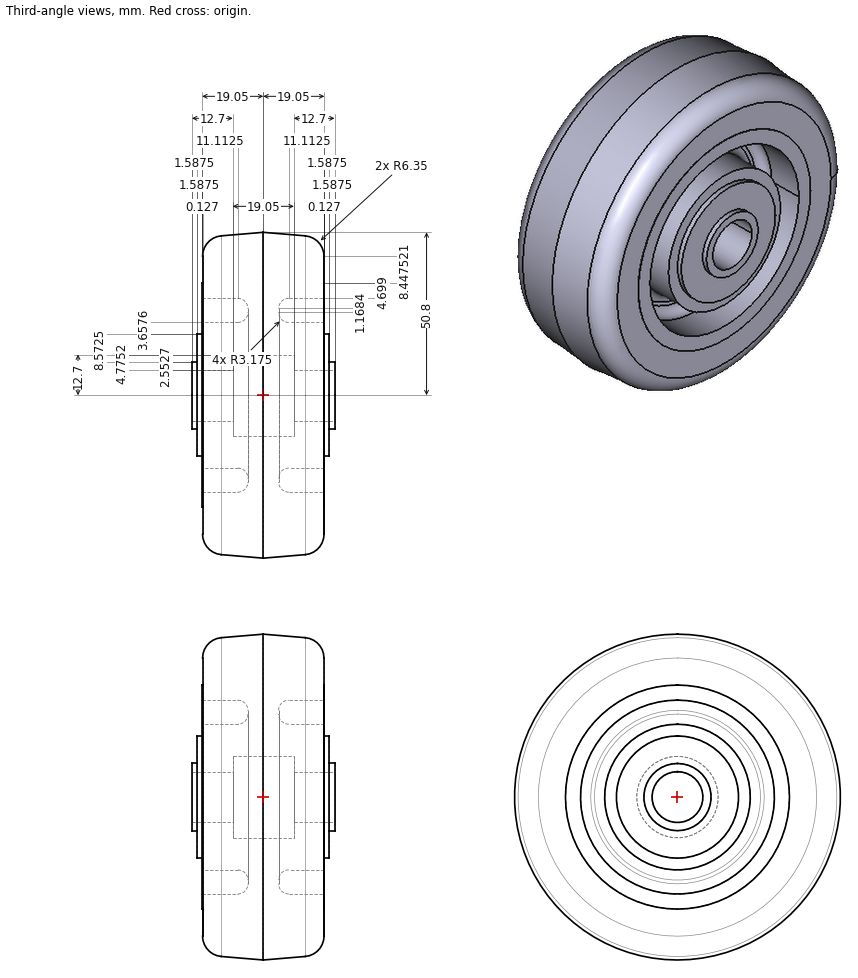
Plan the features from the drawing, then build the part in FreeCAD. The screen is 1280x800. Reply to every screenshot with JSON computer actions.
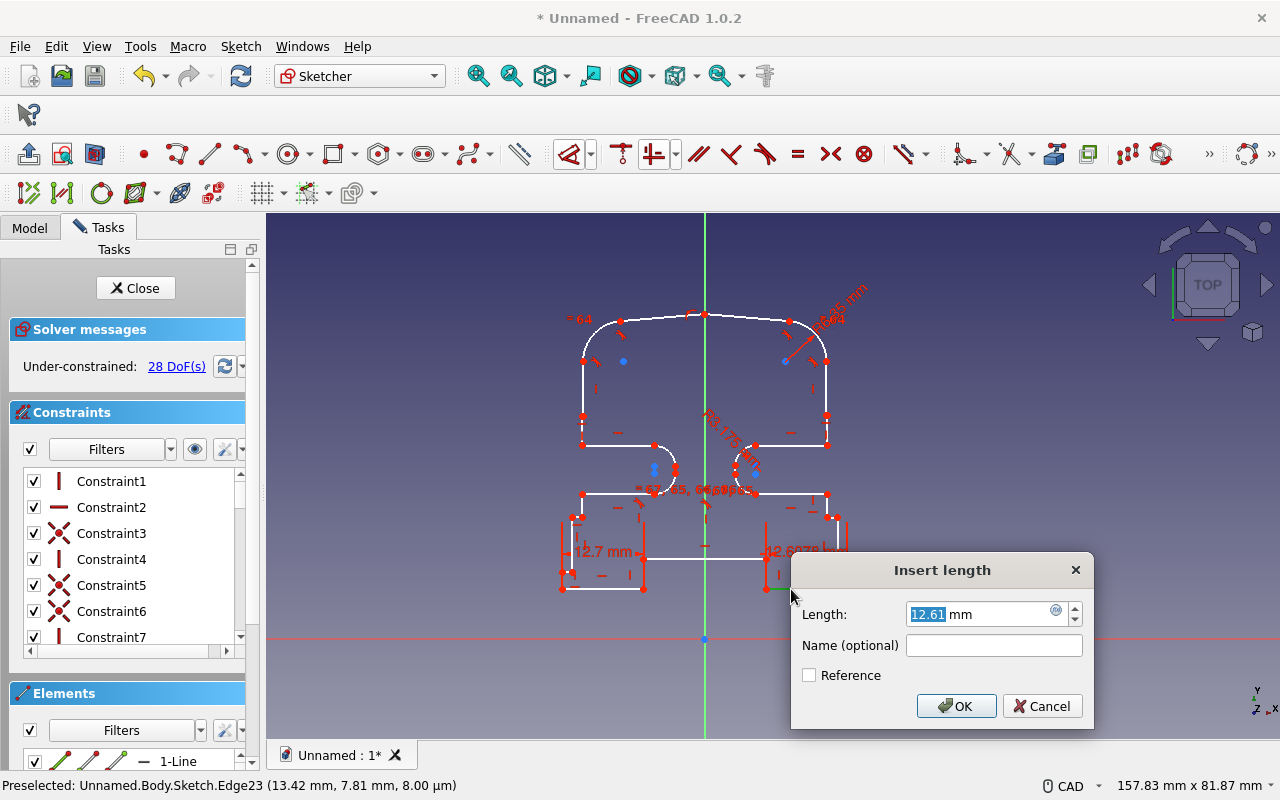
{"action": "type", "text": "12.7"}
{"action": "key", "text": "Return"}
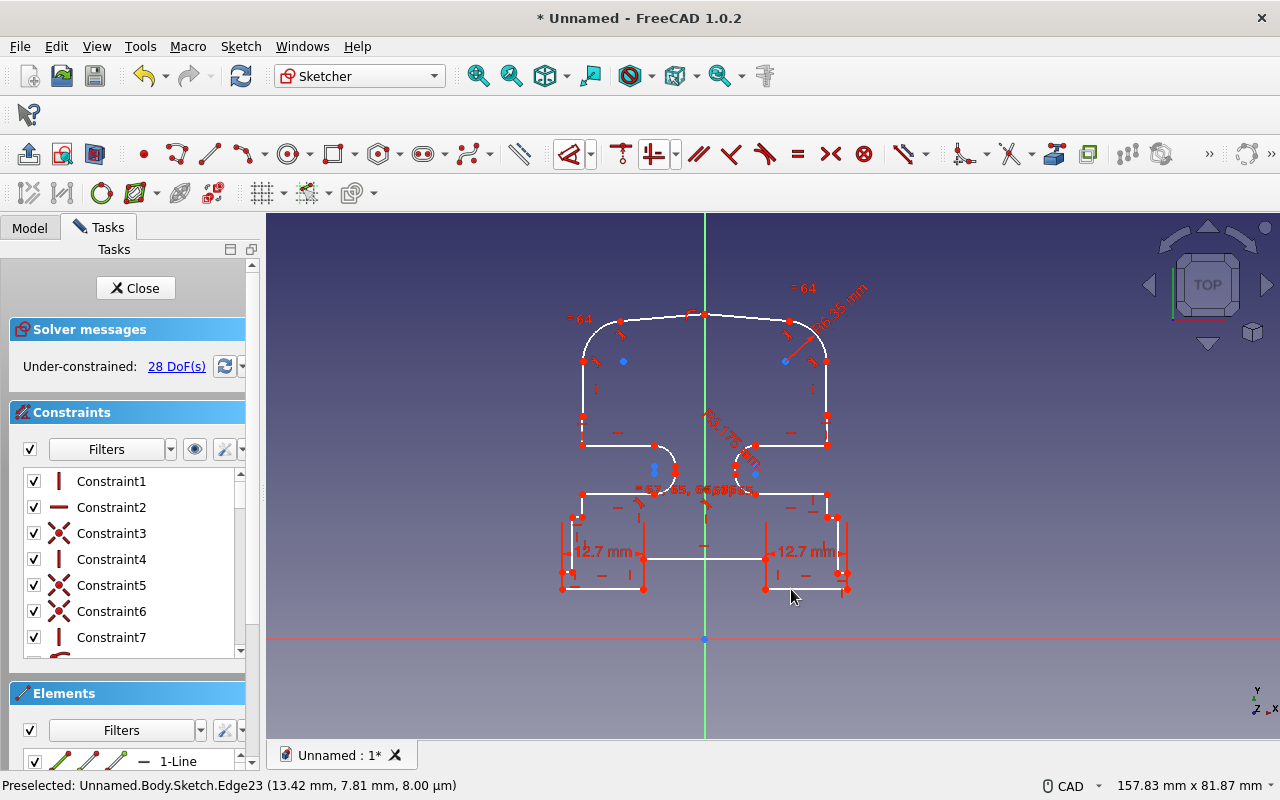
{"action": "scroll", "coordinate": [827, 434], "scroll_direction": "up", "scroll_amount": 2}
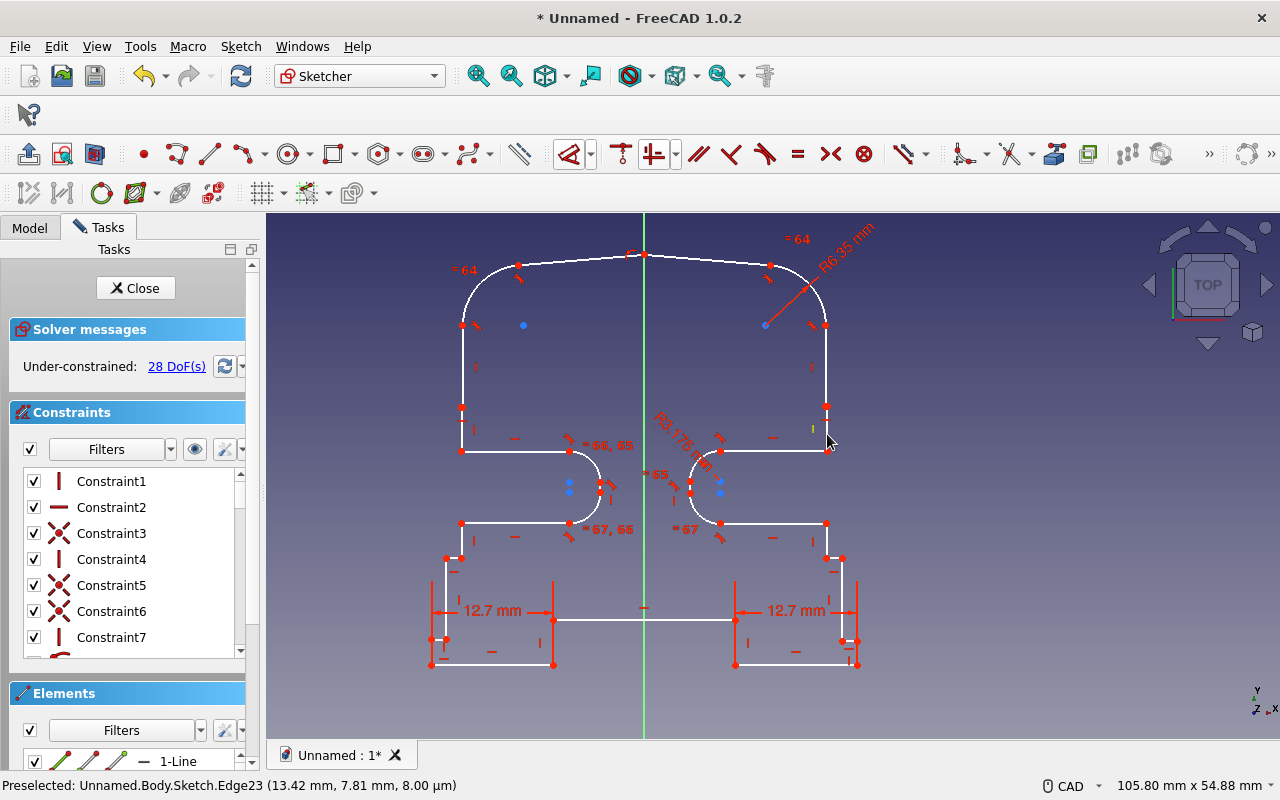
{"action": "left_click", "coordinate": [827, 433]}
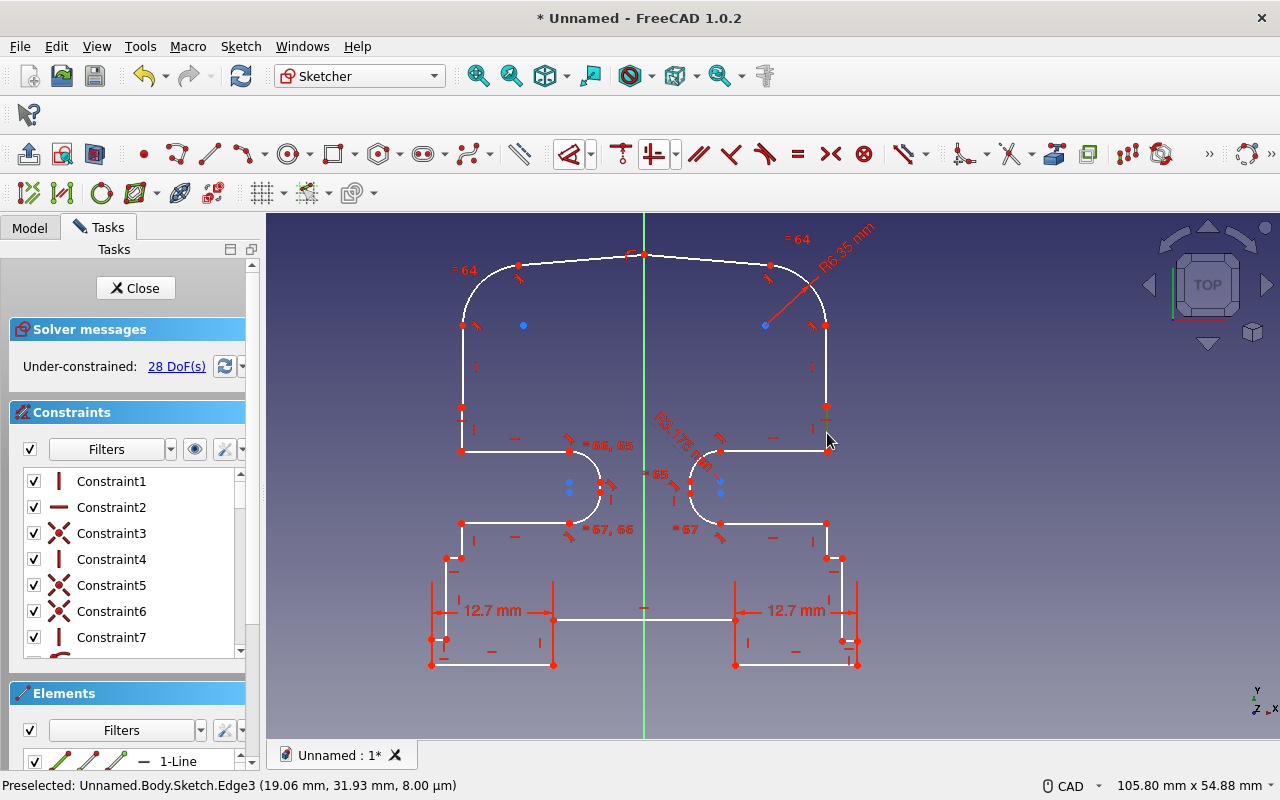
{"action": "key", "text": "i"}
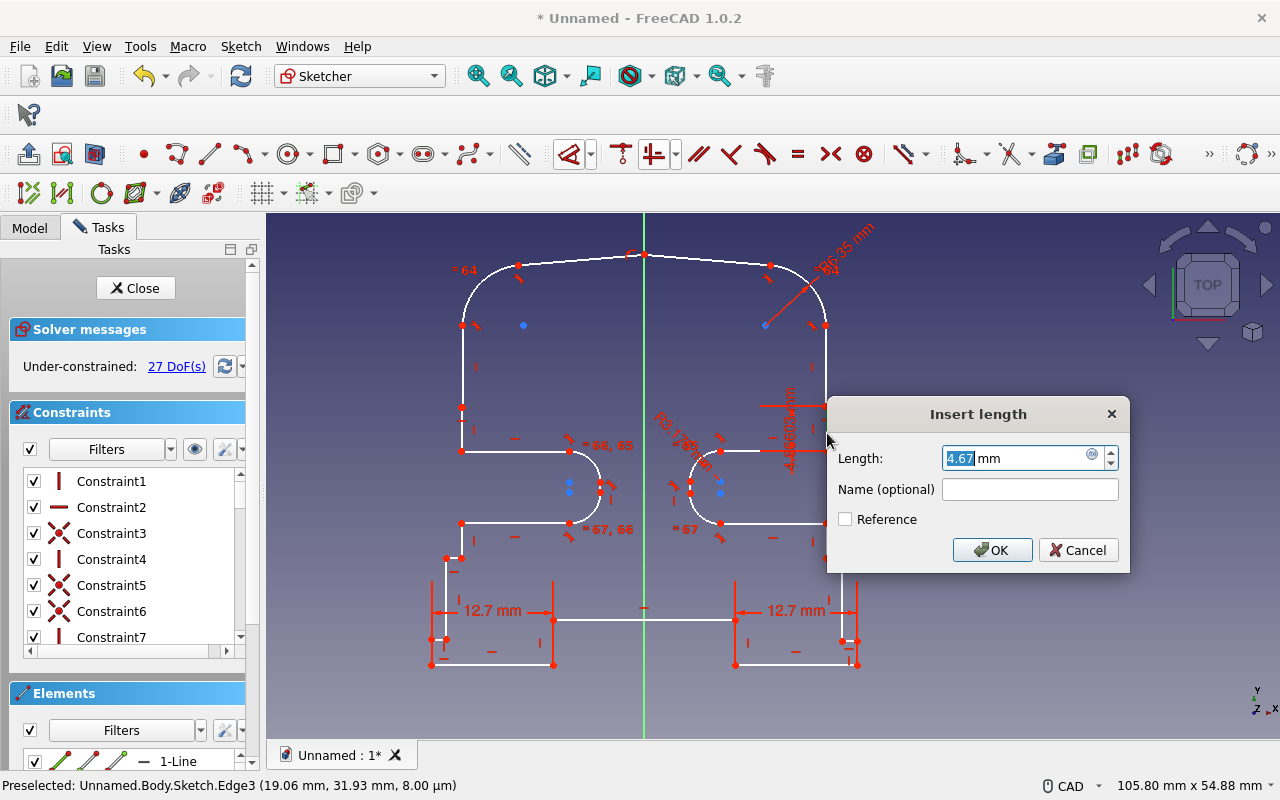
{"action": "type", "text": "4.699"}
{"action": "key", "text": "Return"}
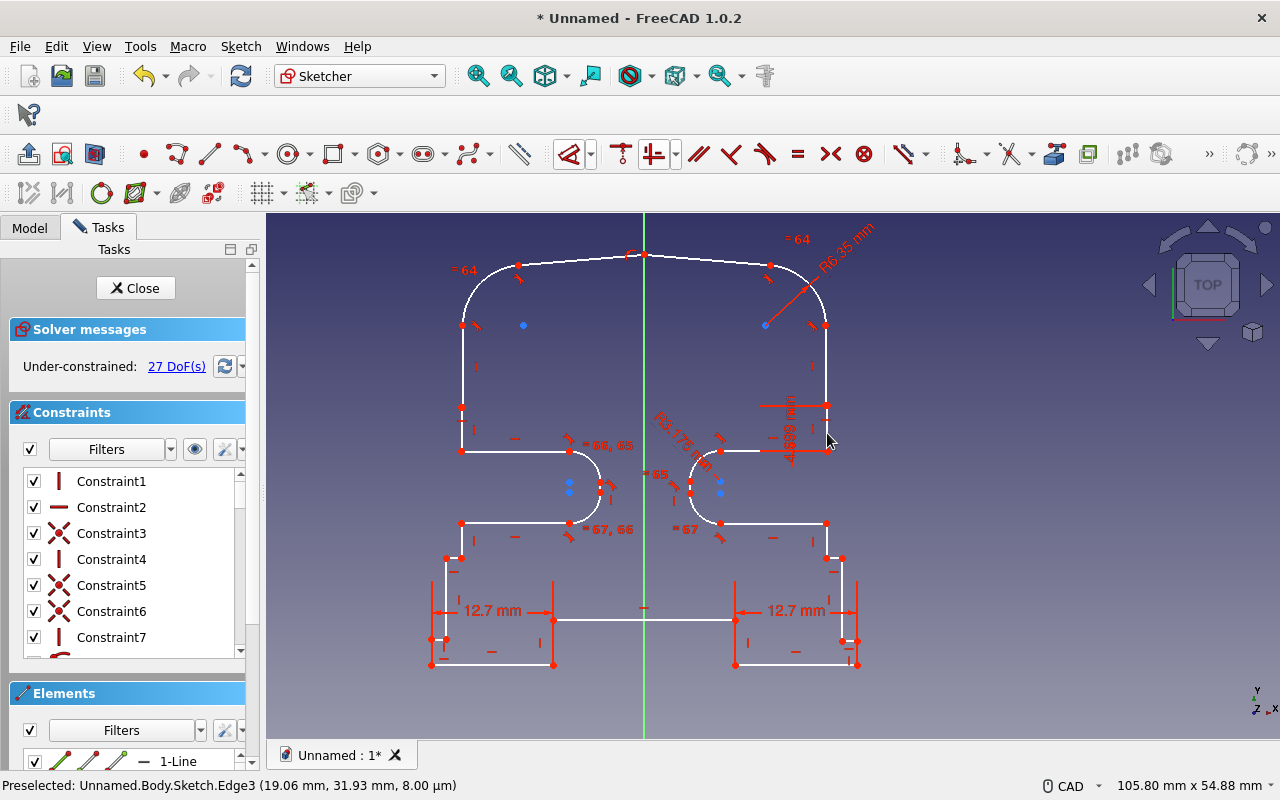
{"action": "scroll", "coordinate": [826, 406], "scroll_direction": "up", "scroll_amount": 18}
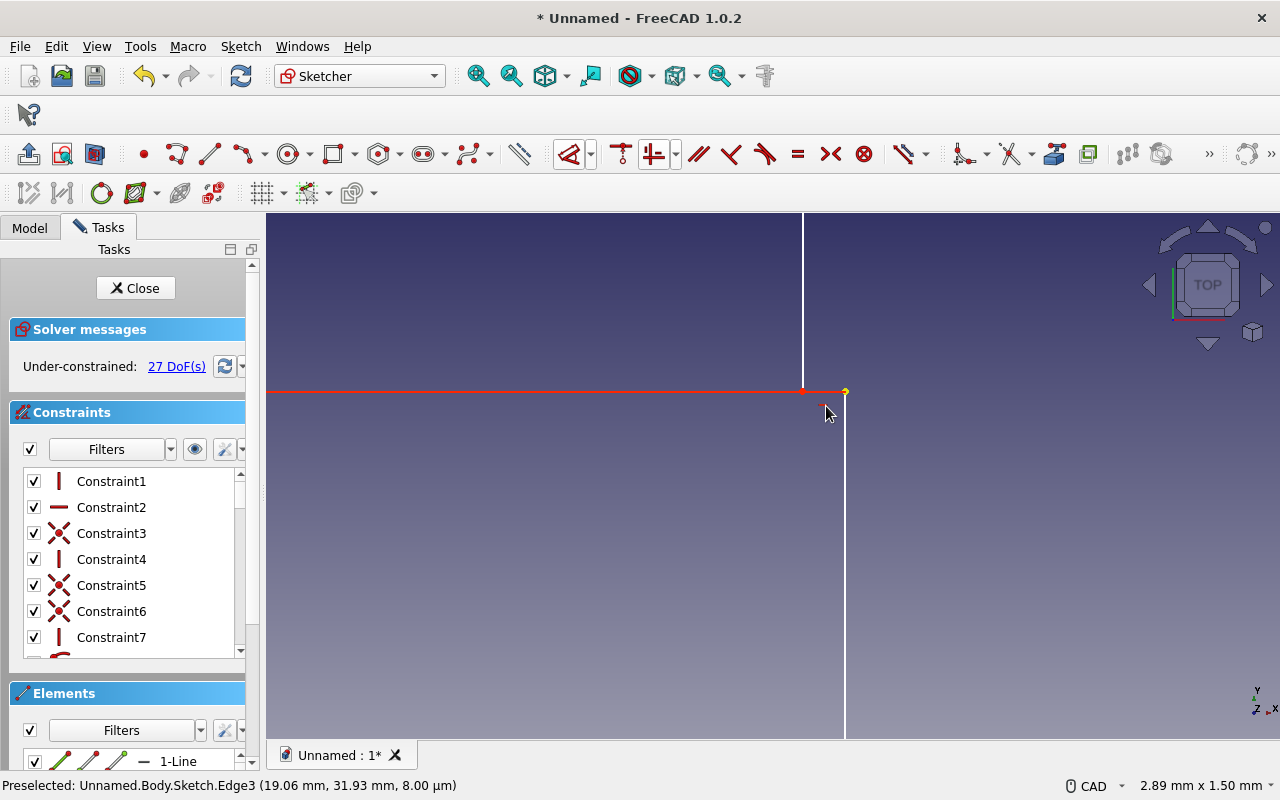
{"action": "left_click", "coordinate": [824, 392]}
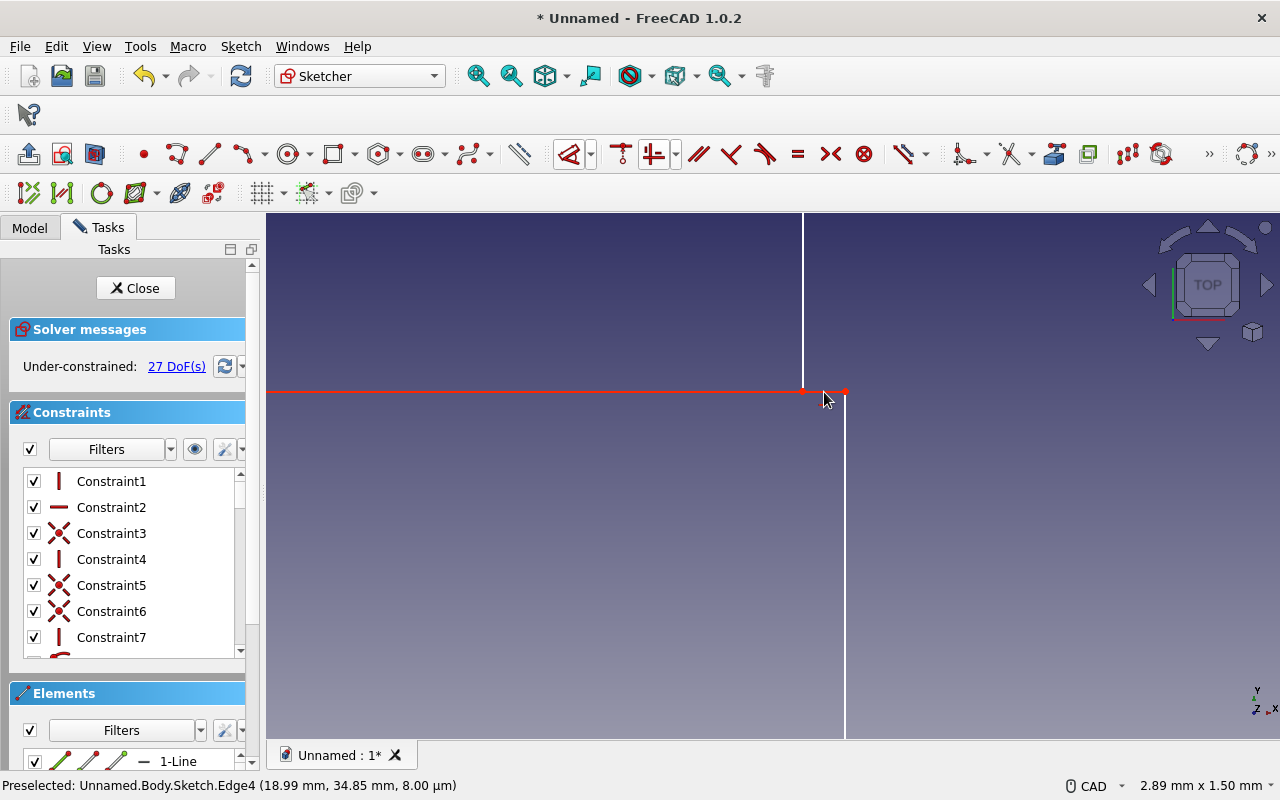
{"action": "left_click", "coordinate": [590, 154]}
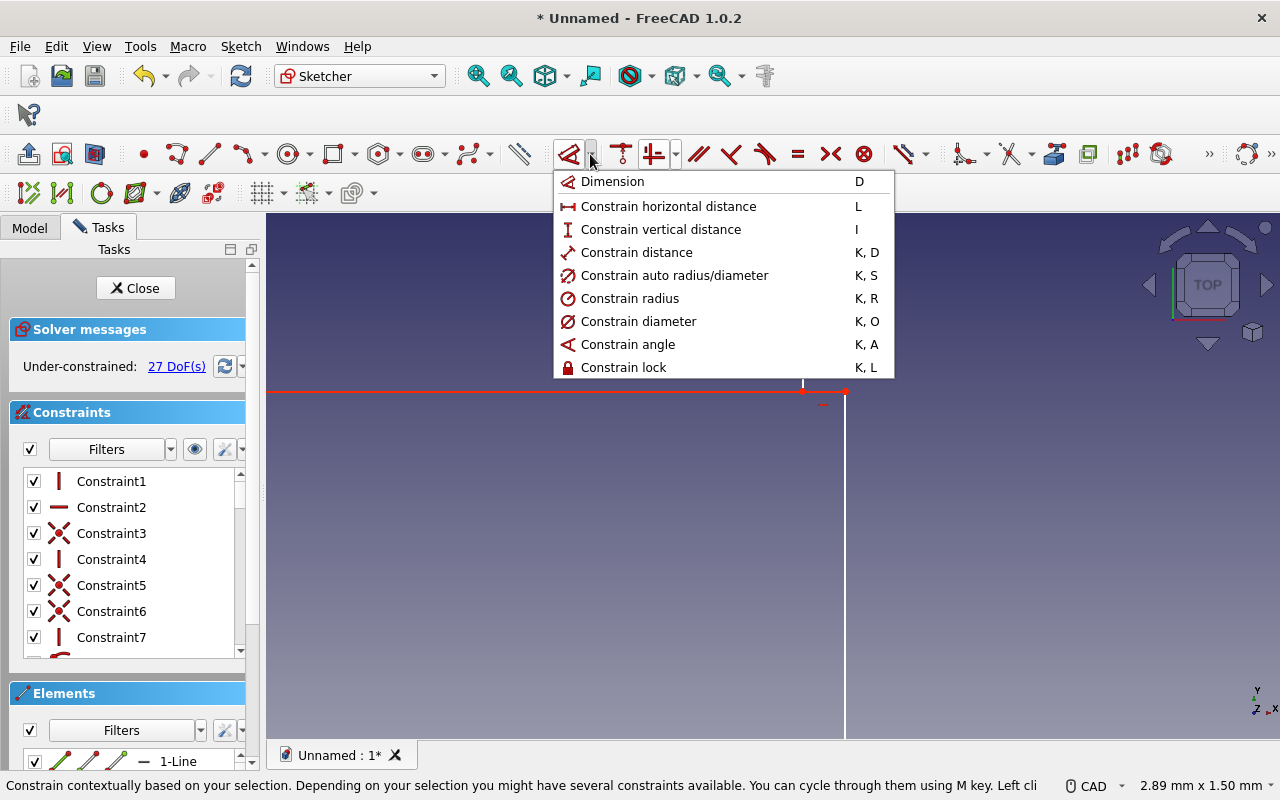
{"action": "left_click", "coordinate": [724, 206]}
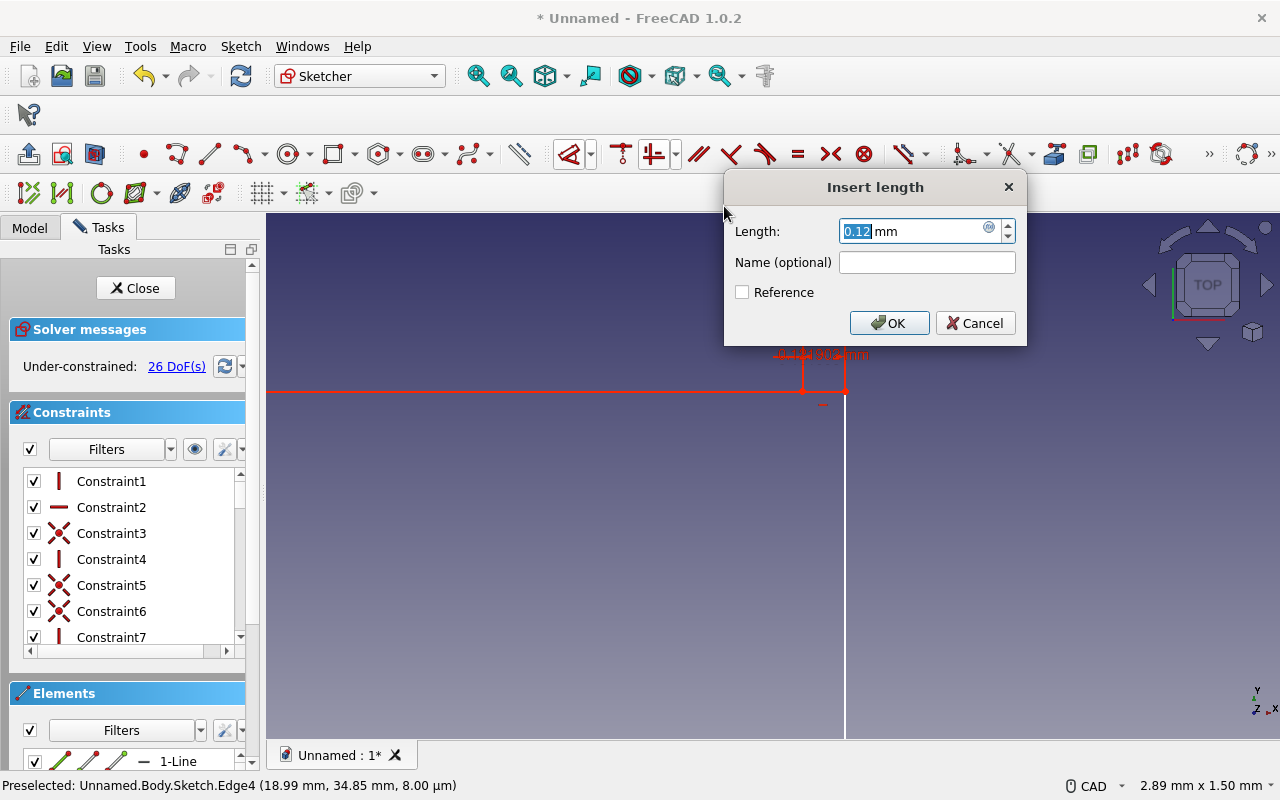
{"action": "type", "text": "0.127"}
{"action": "key", "text": "Return"}